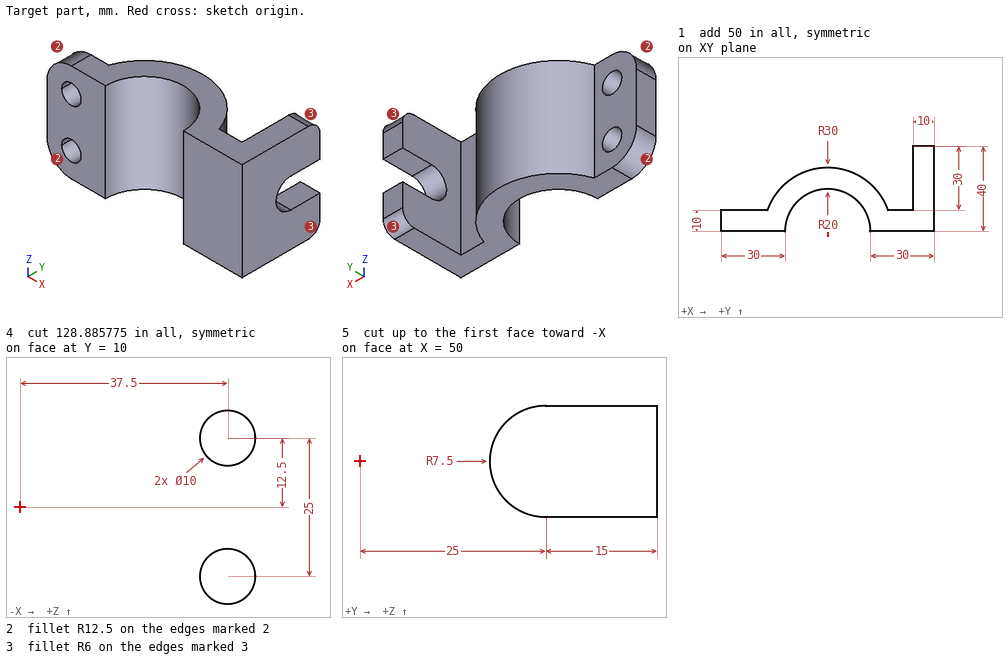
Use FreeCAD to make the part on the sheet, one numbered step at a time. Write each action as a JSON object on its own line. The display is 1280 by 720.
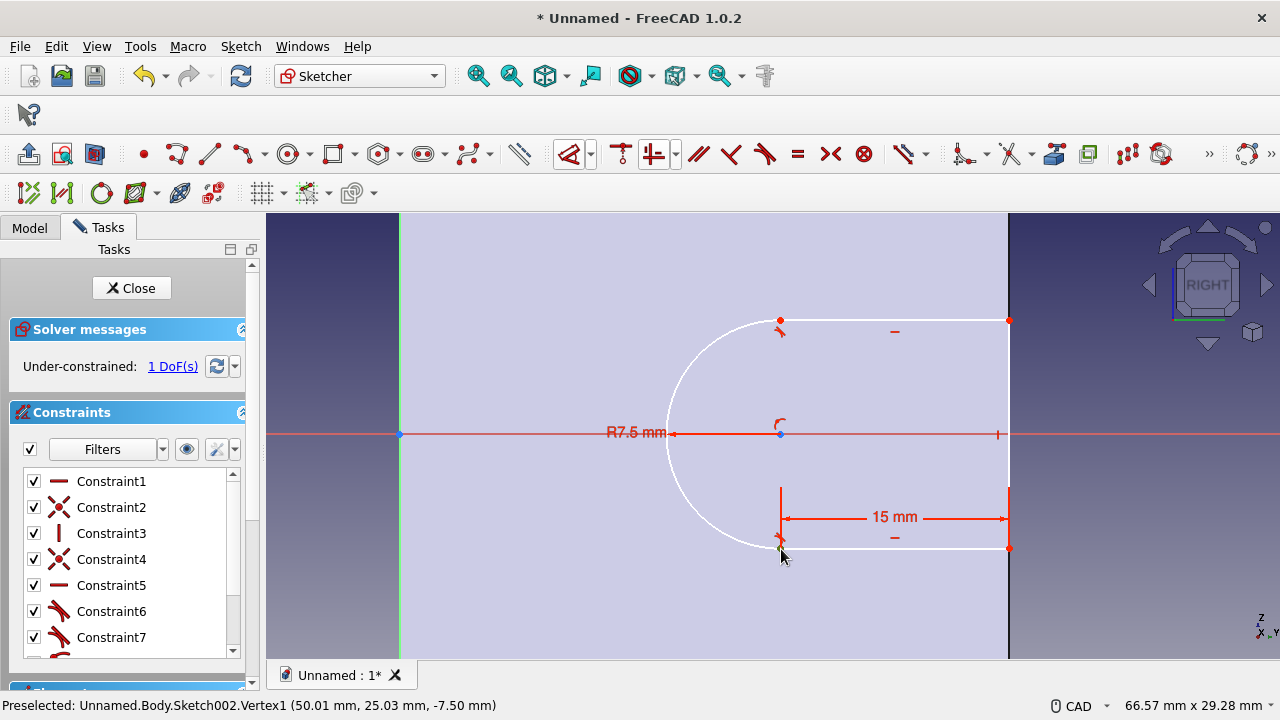
{"action": "left_click", "coordinate": [590, 154]}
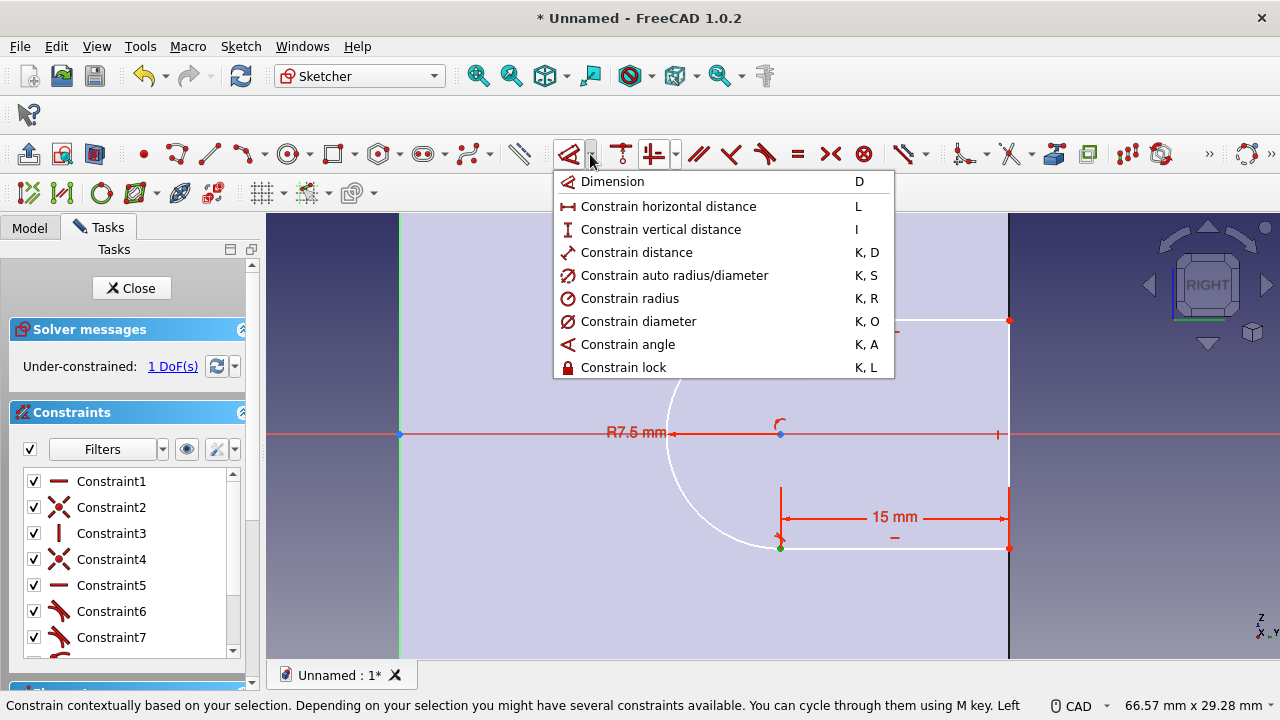
{"action": "left_click", "coordinate": [724, 206]}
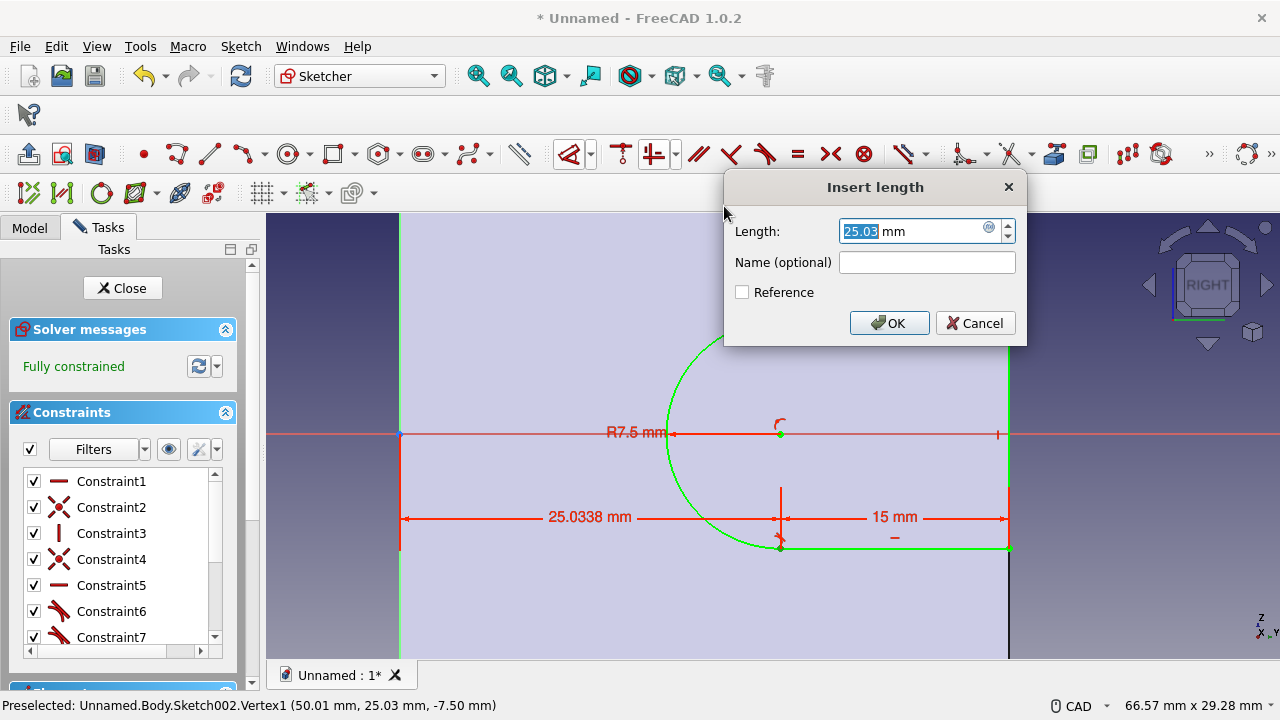
{"action": "type", "text": "25"}
{"action": "key", "text": "Return"}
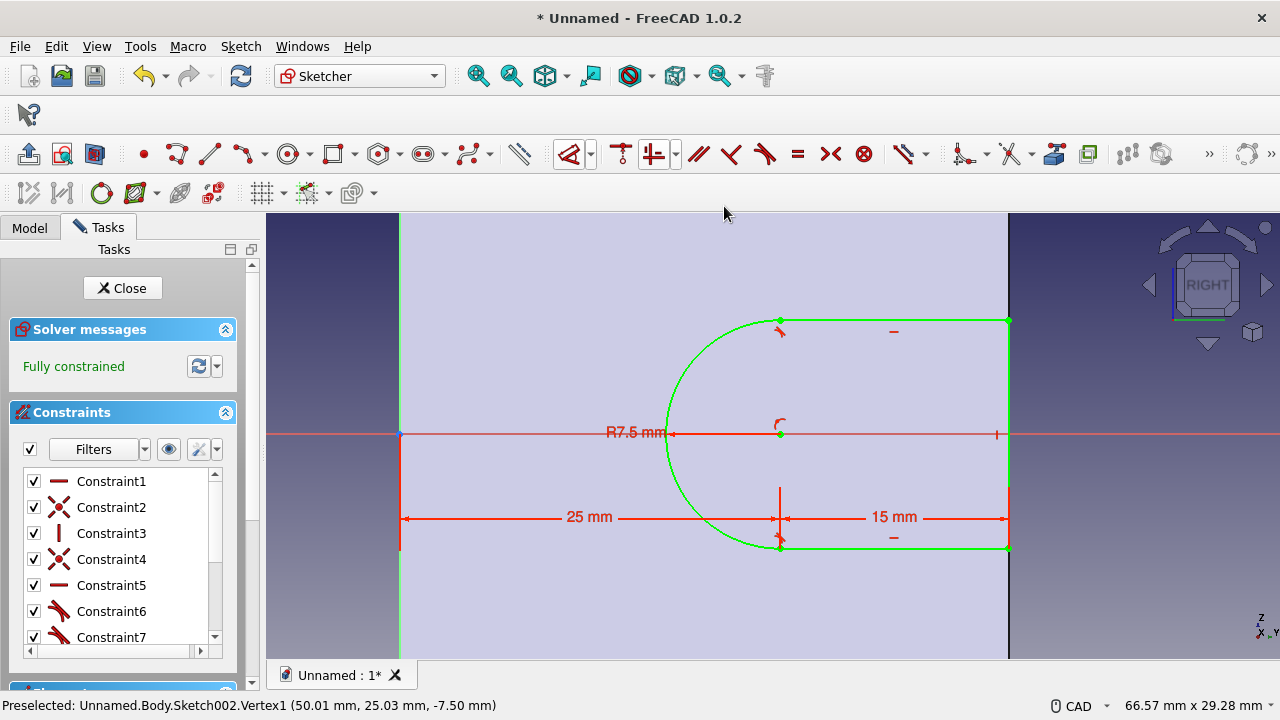
{"action": "left_click", "coordinate": [123, 288]}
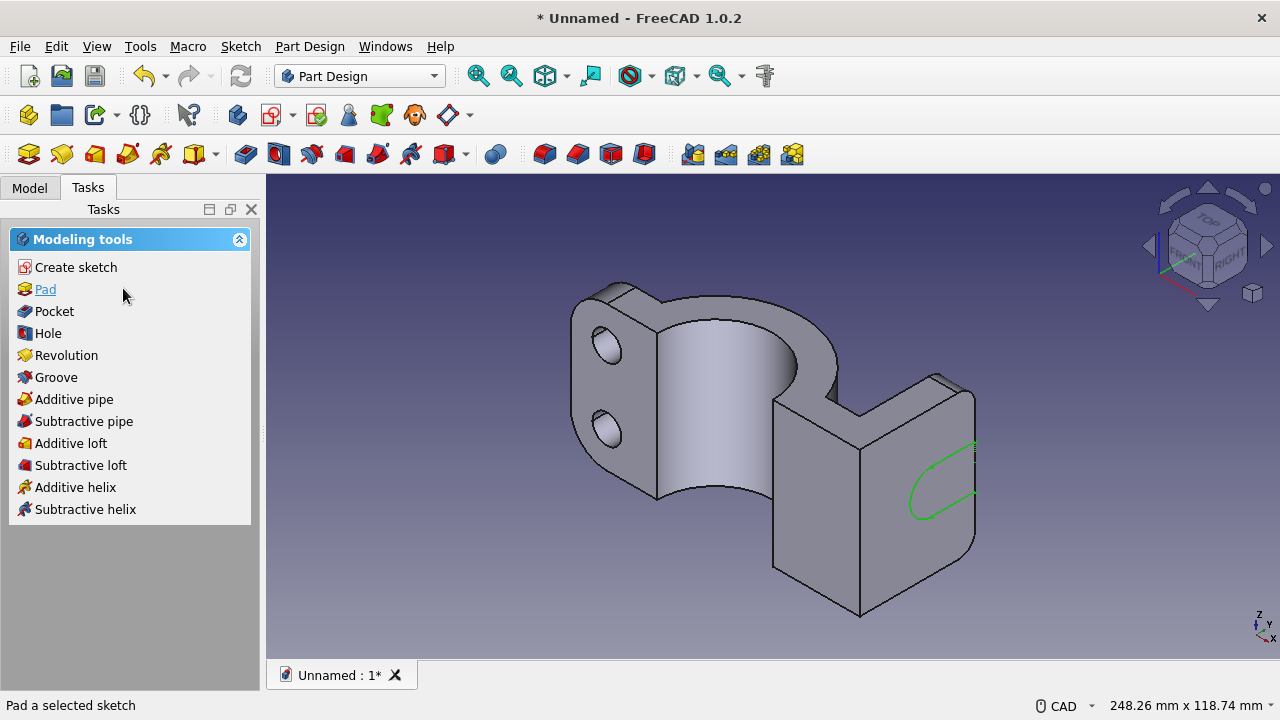
{"action": "left_click", "coordinate": [246, 154]}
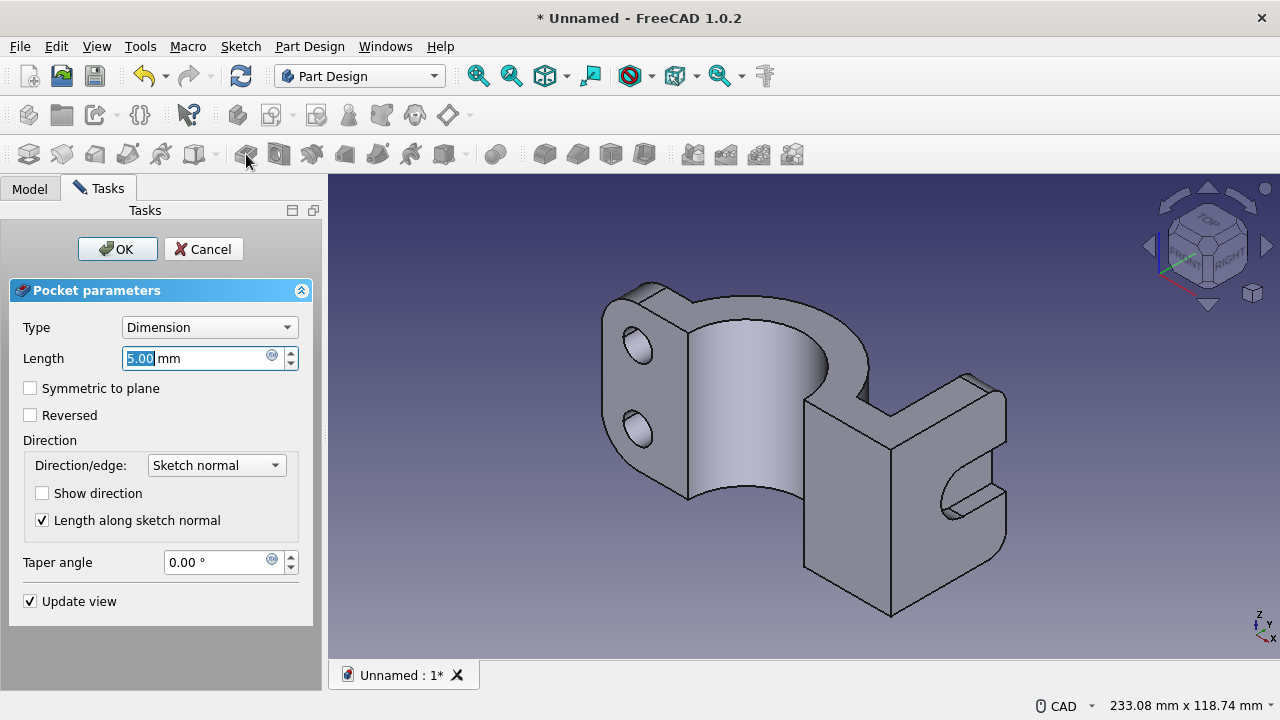
{"action": "left_click", "coordinate": [210, 328]}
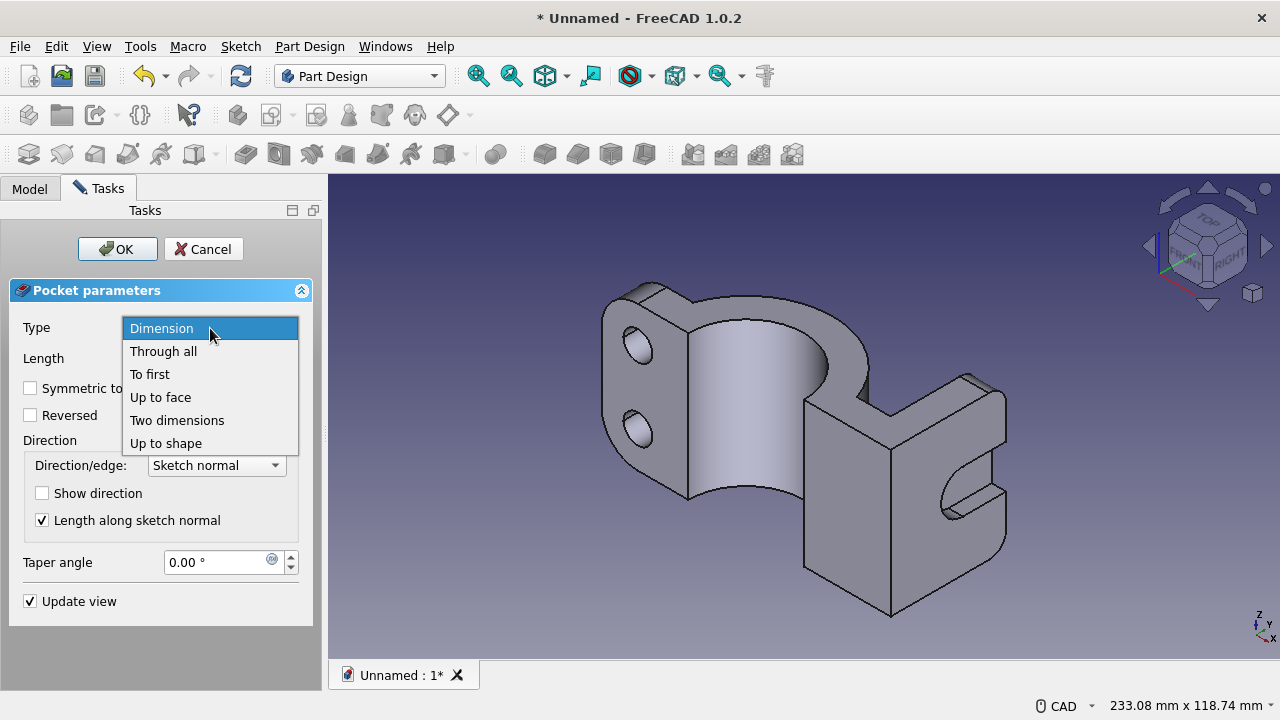
{"action": "left_click", "coordinate": [208, 374]}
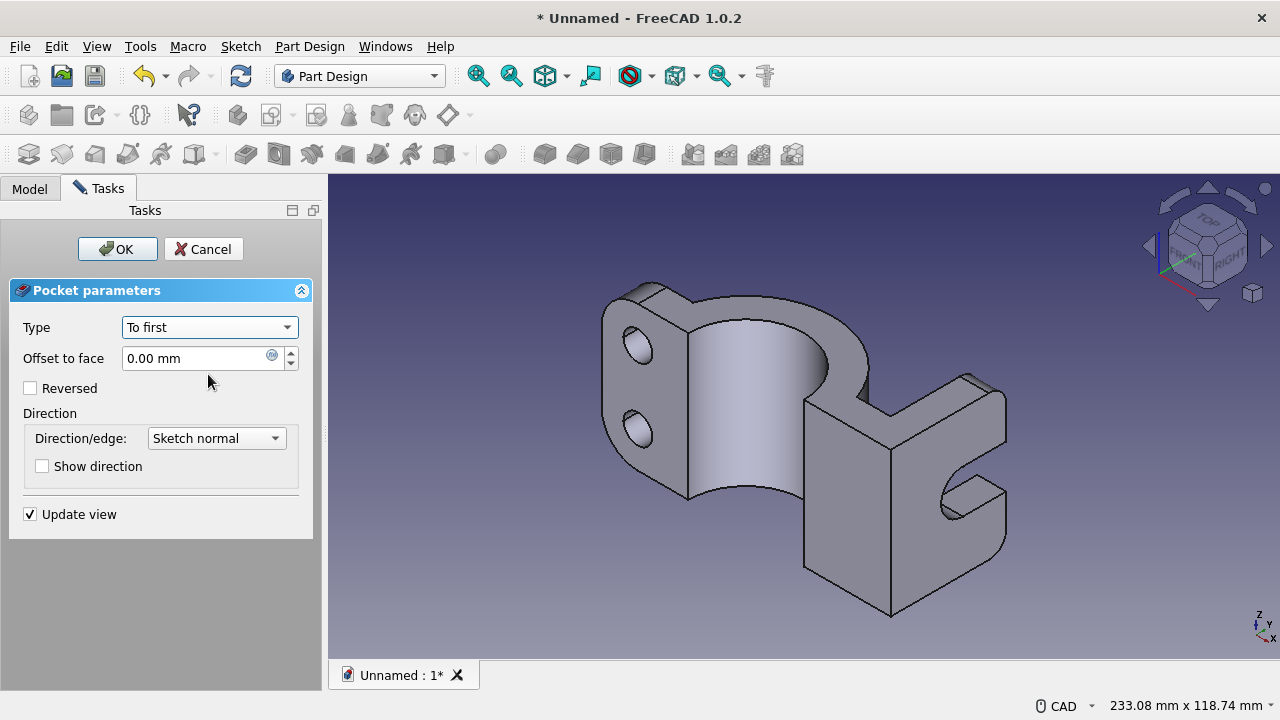
{"action": "left_click", "coordinate": [118, 249]}